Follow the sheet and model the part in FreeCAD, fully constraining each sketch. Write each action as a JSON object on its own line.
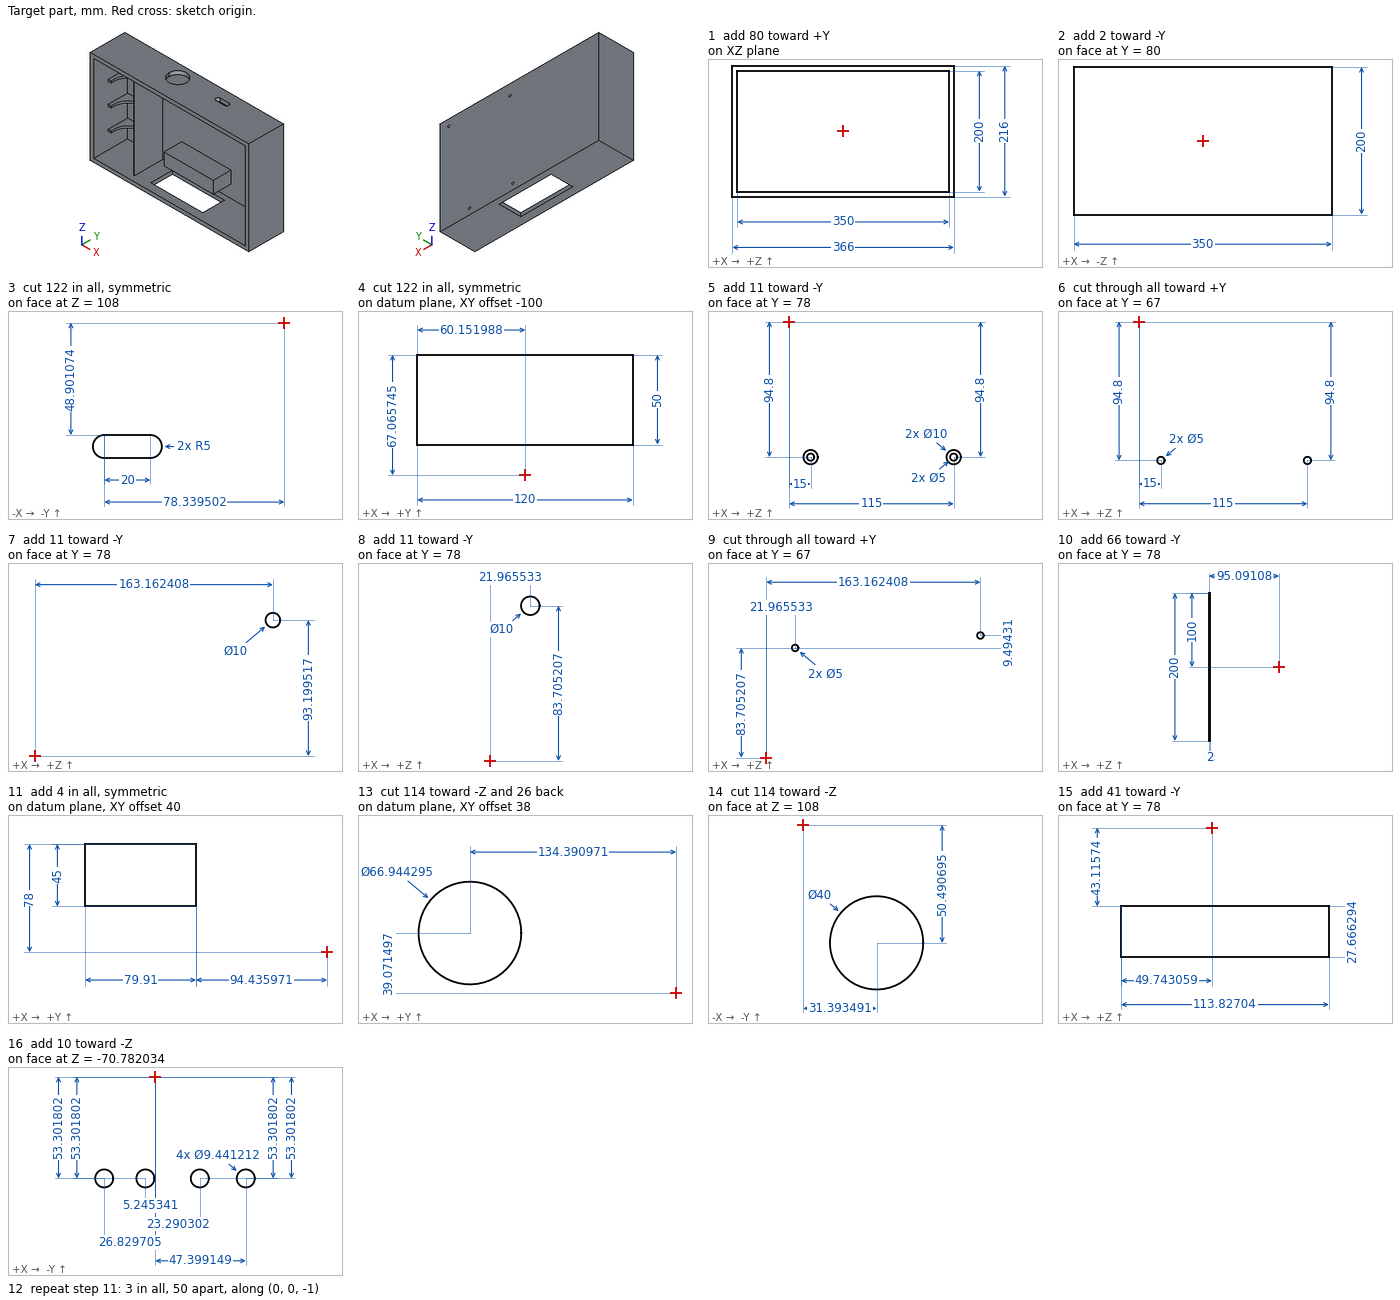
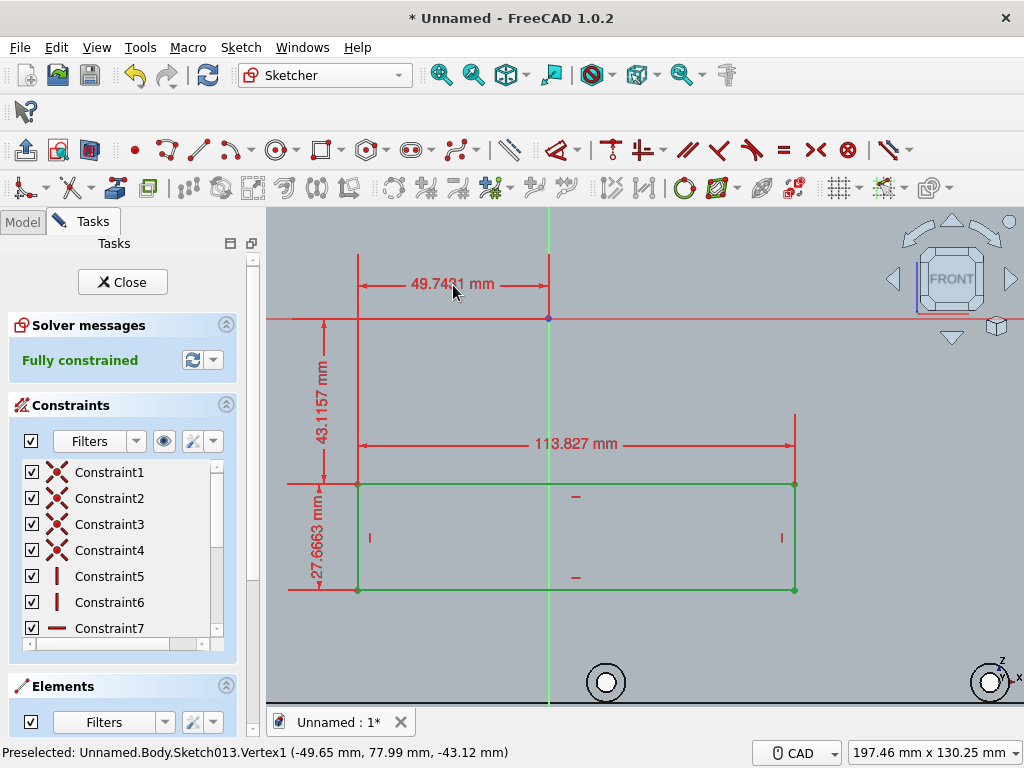
{"action": "left_click", "coordinate": [123, 282]}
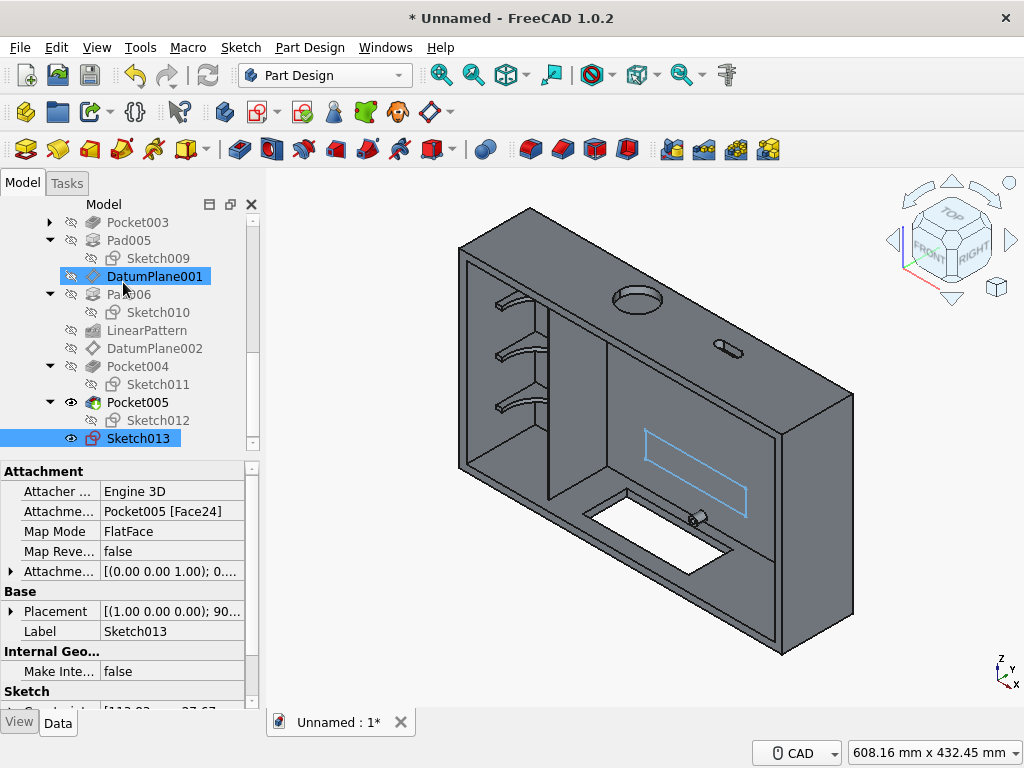
{"action": "left_click", "coordinate": [26, 150]}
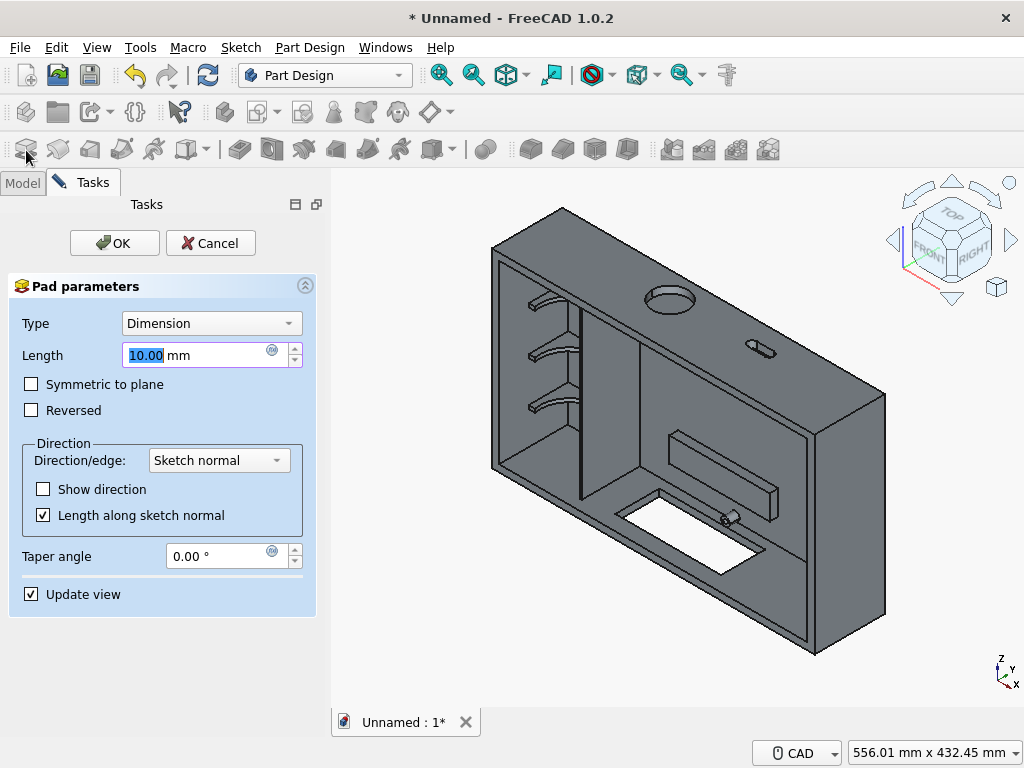
{"action": "type", "text": "41"}
{"action": "key", "text": "Tab"}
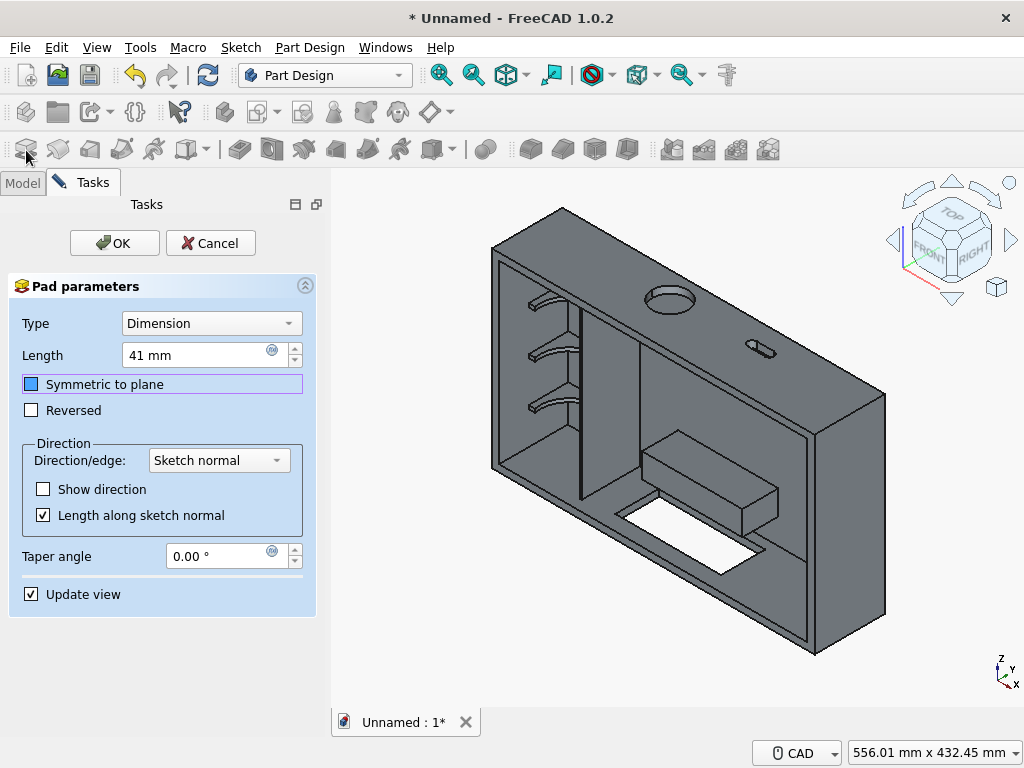
{"action": "left_click", "coordinate": [115, 243]}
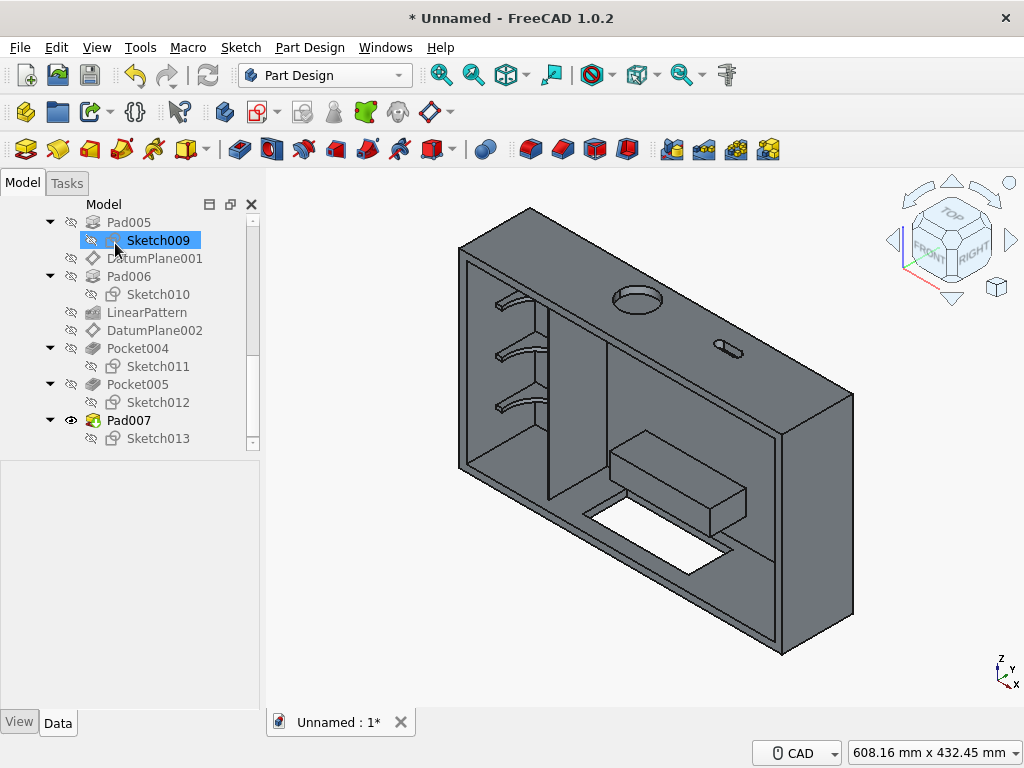
{"action": "key", "text": "5"}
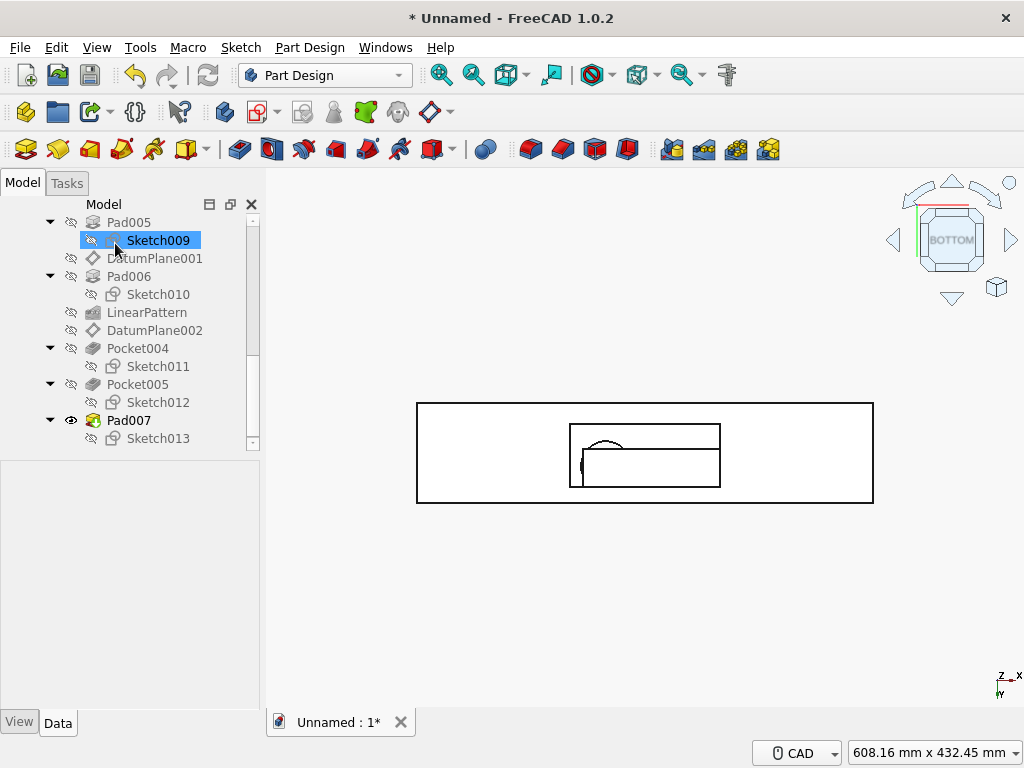
{"action": "left_click", "coordinate": [694, 474]}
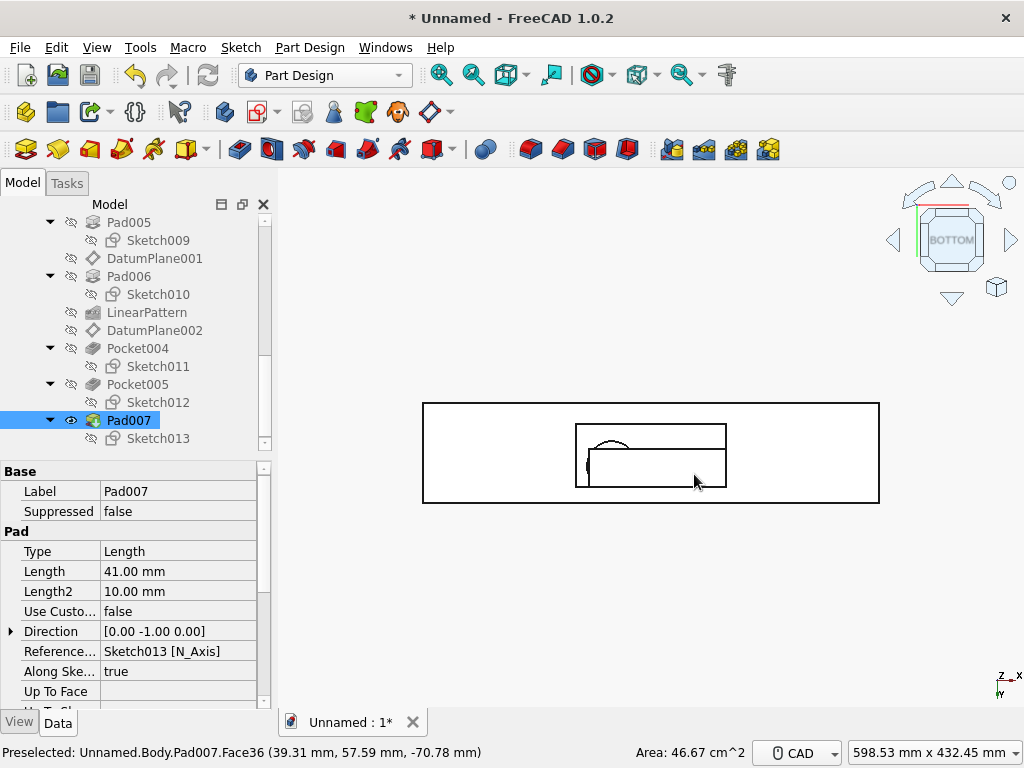
{"action": "left_click", "coordinate": [258, 112]}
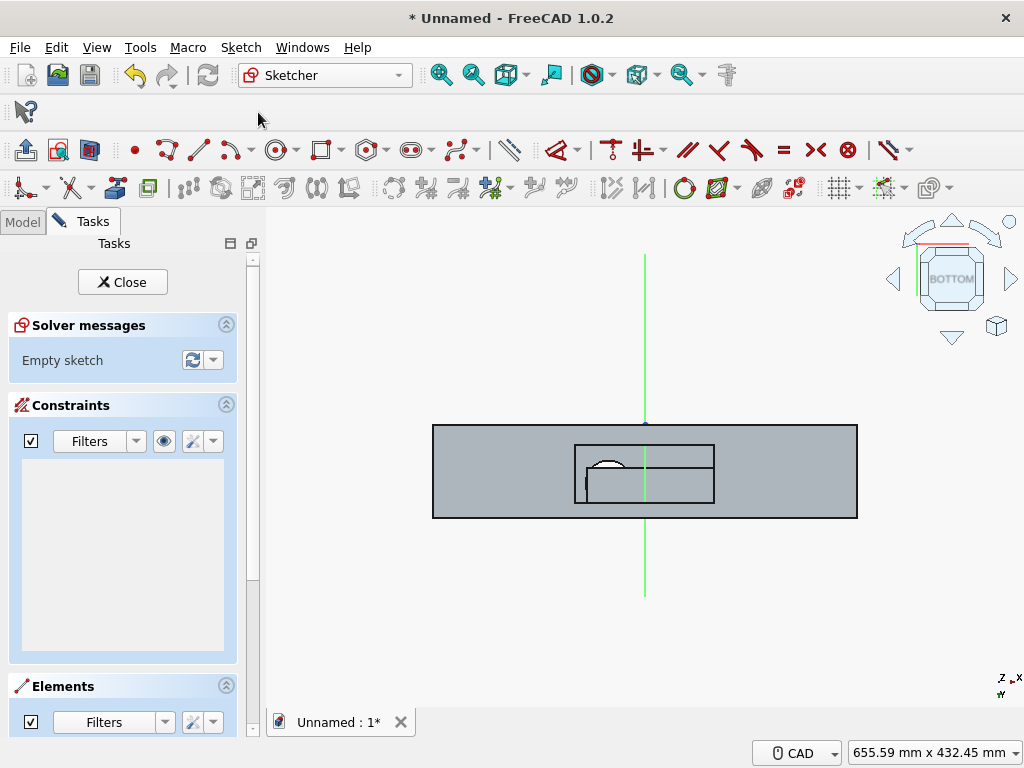
{"action": "scroll", "coordinate": [683, 459], "scroll_direction": "up", "scroll_amount": 7}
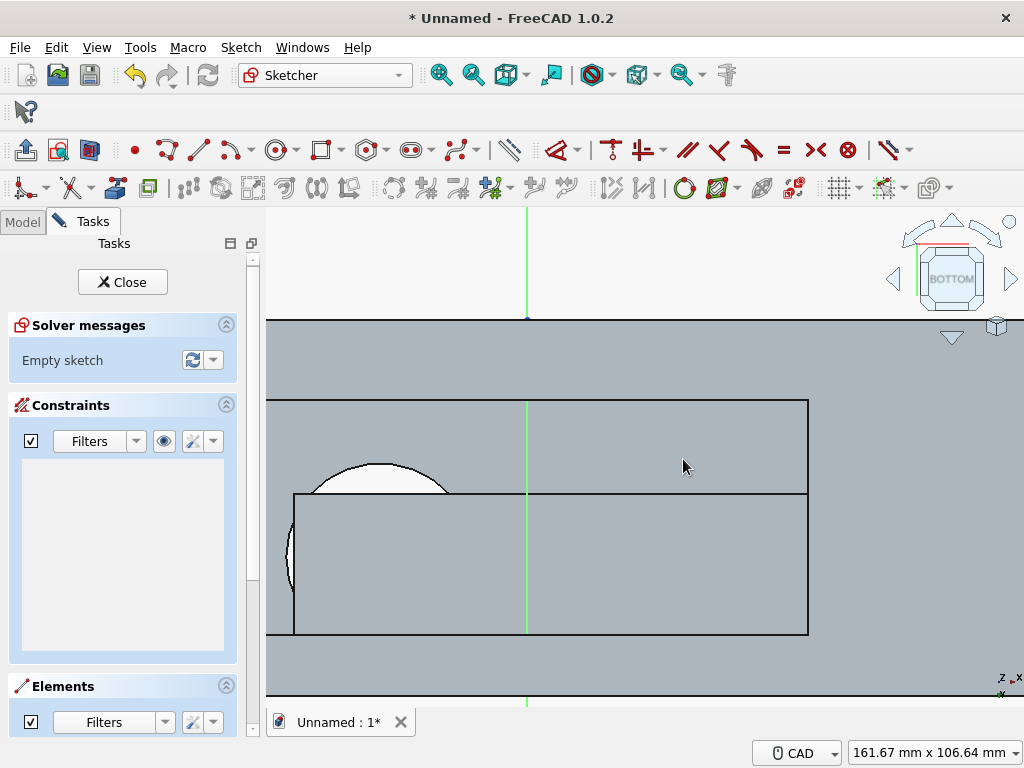
{"action": "left_click", "coordinate": [276, 150]}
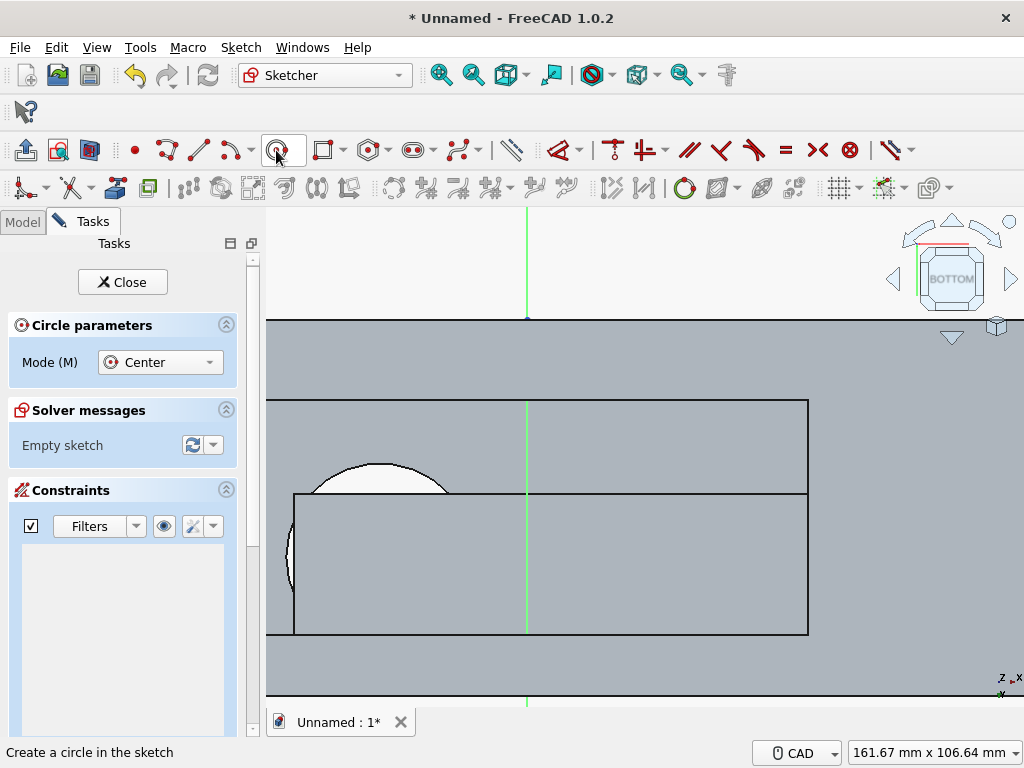
{"action": "left_click", "coordinate": [749, 570]}
{"action": "mouse_move", "coordinate": [765, 555]}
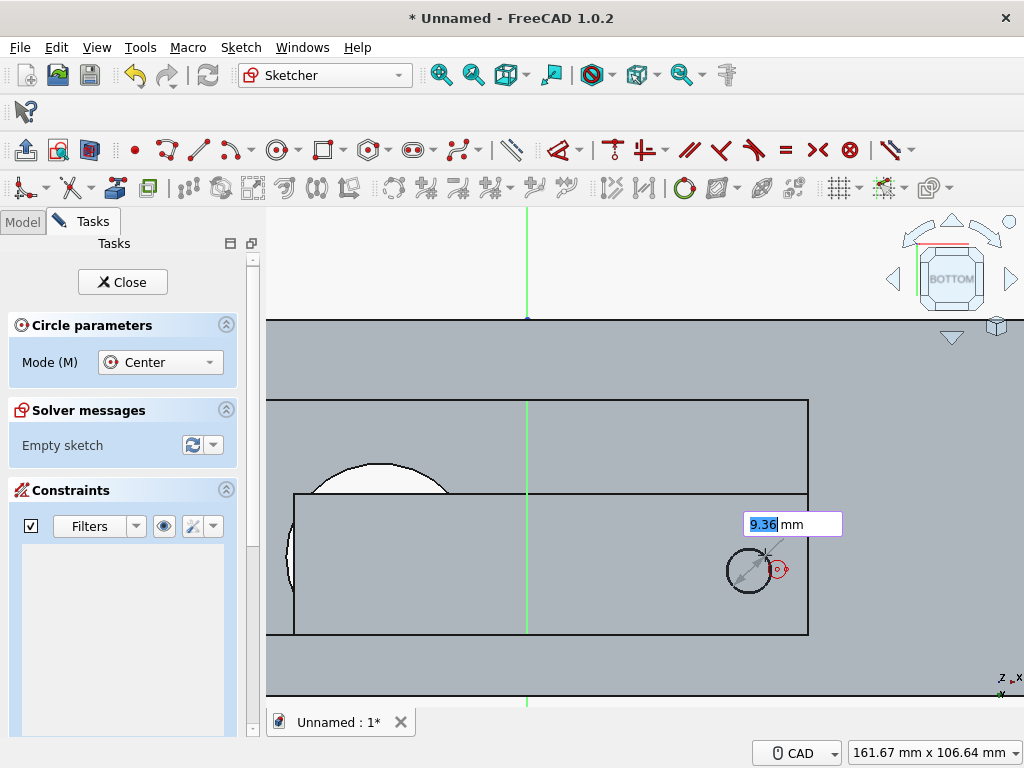
{"action": "type", "text": "9.441212"}
{"action": "key", "text": "Return"}